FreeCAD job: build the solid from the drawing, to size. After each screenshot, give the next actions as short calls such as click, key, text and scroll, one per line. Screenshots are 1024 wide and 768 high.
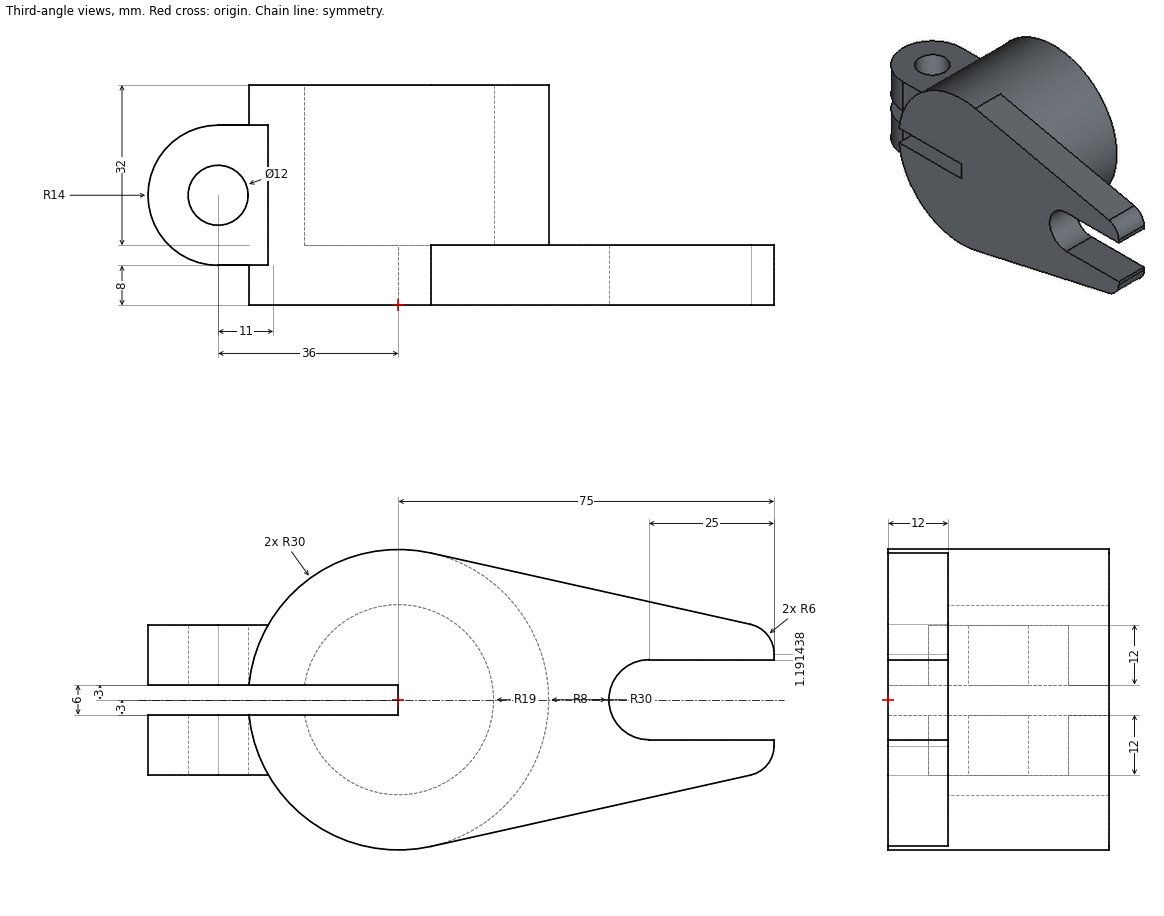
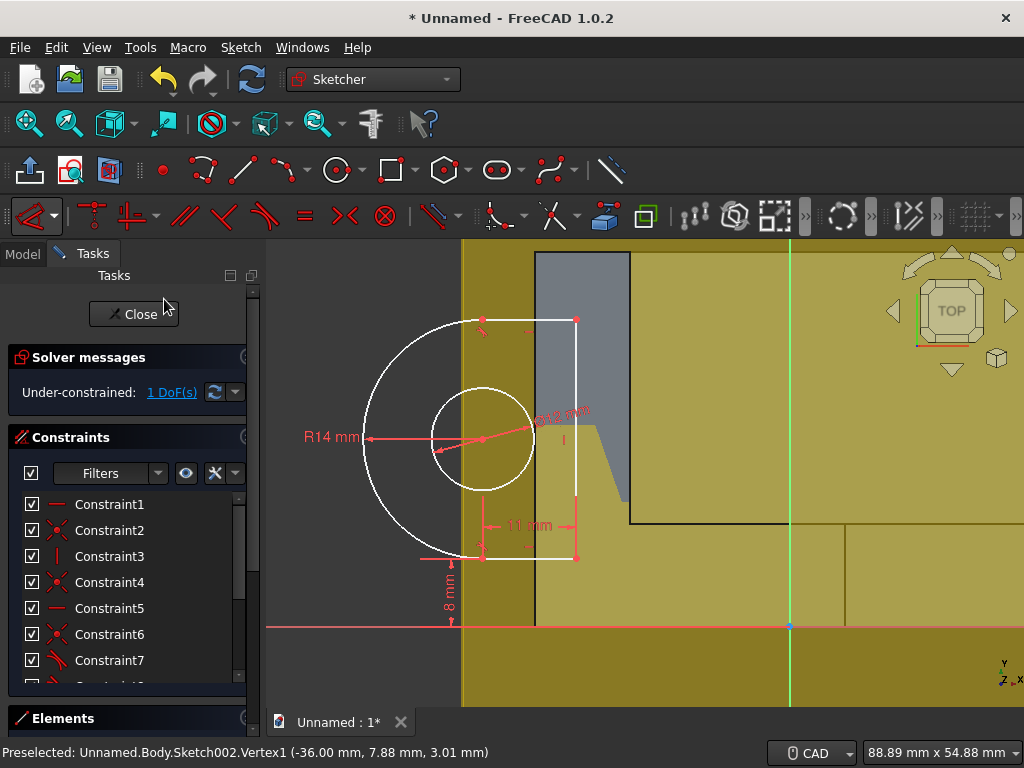
click(483, 439)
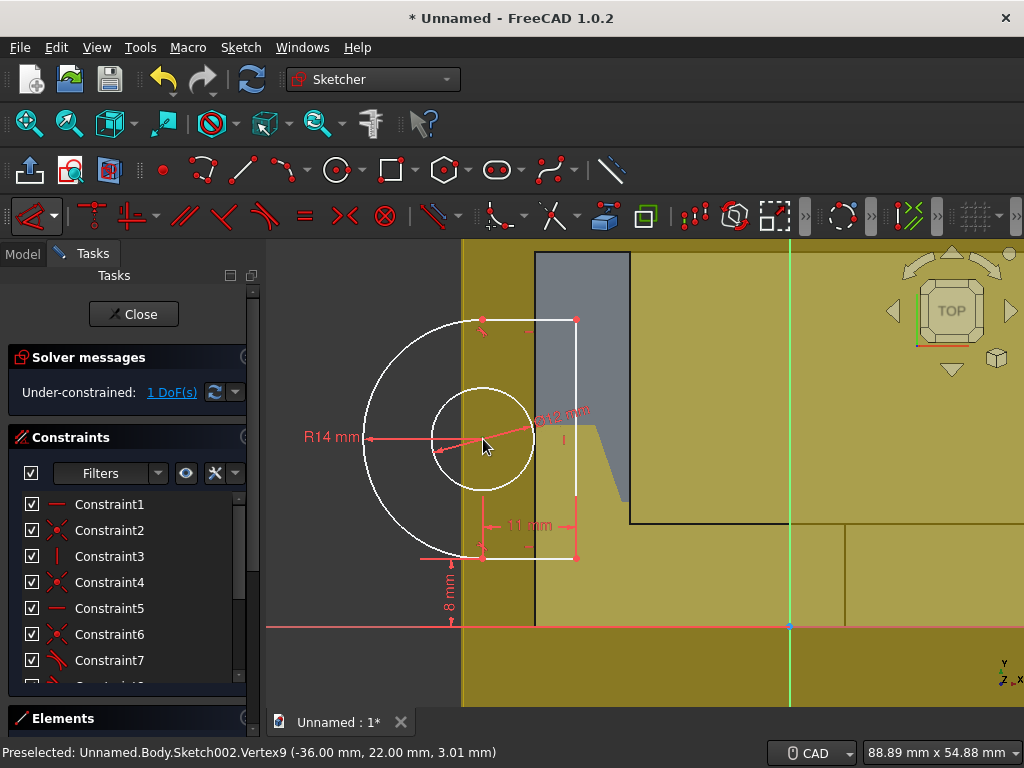
key(l)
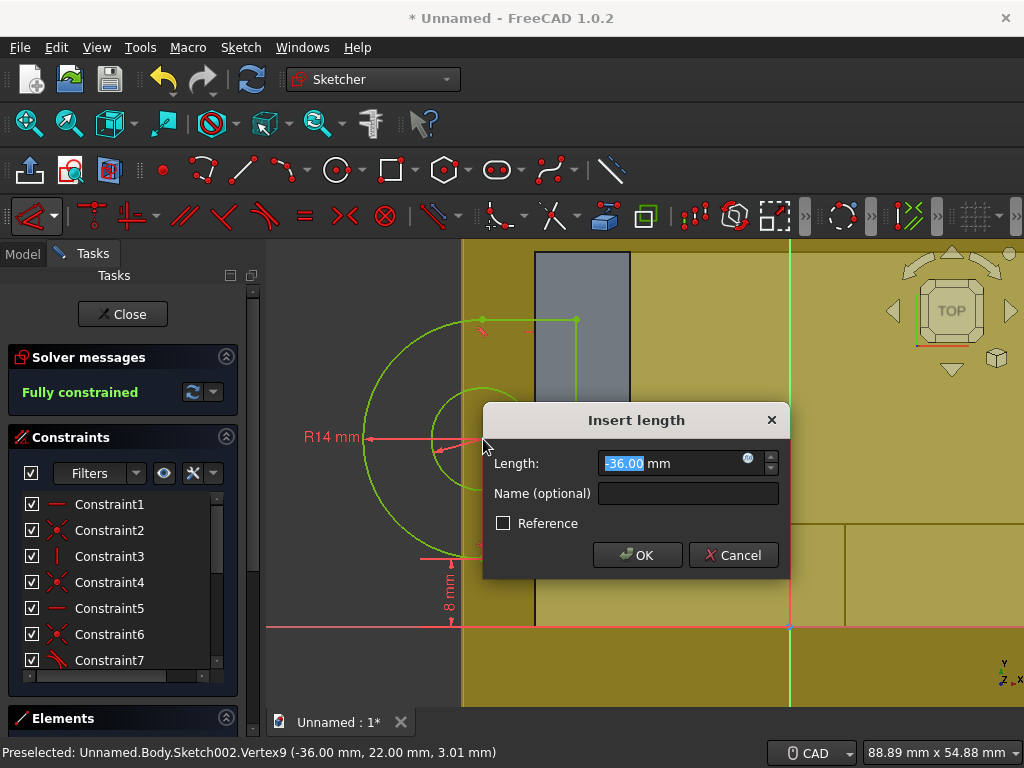
text(-36)
key(Return)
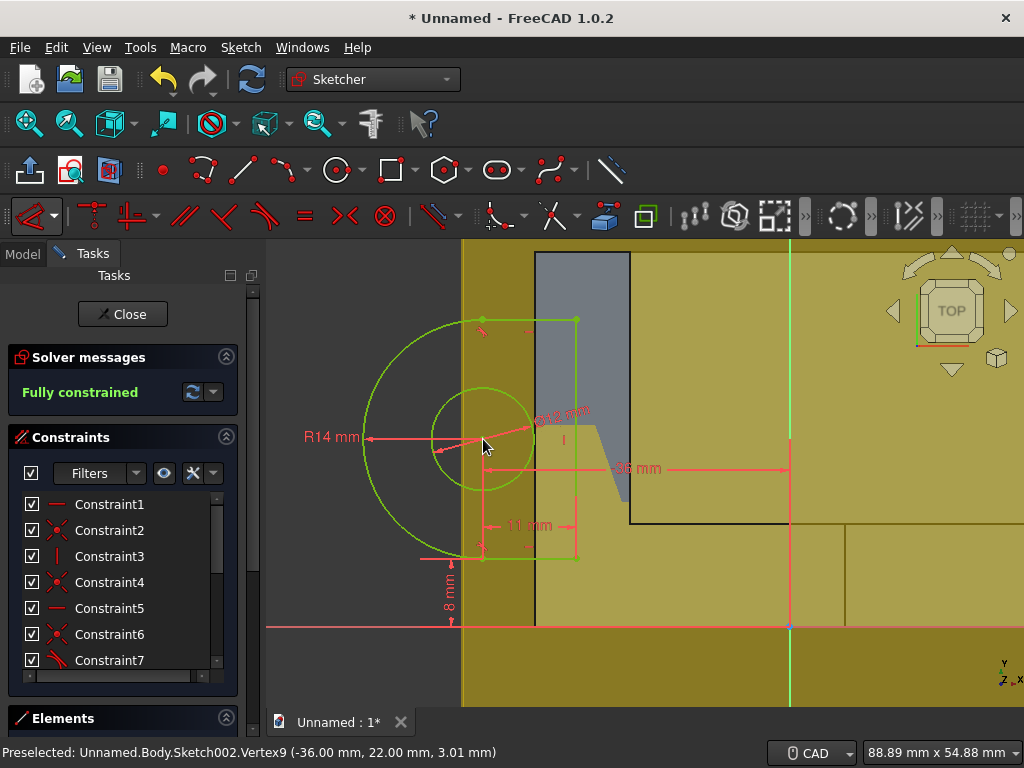
click(123, 314)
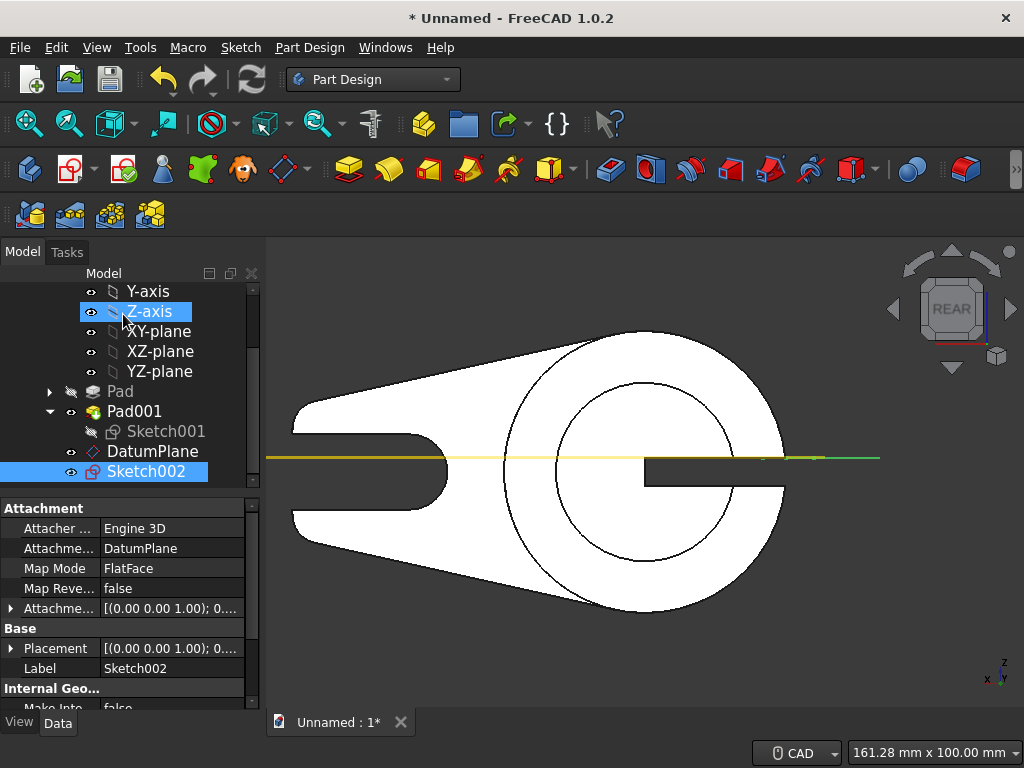
click(350, 170)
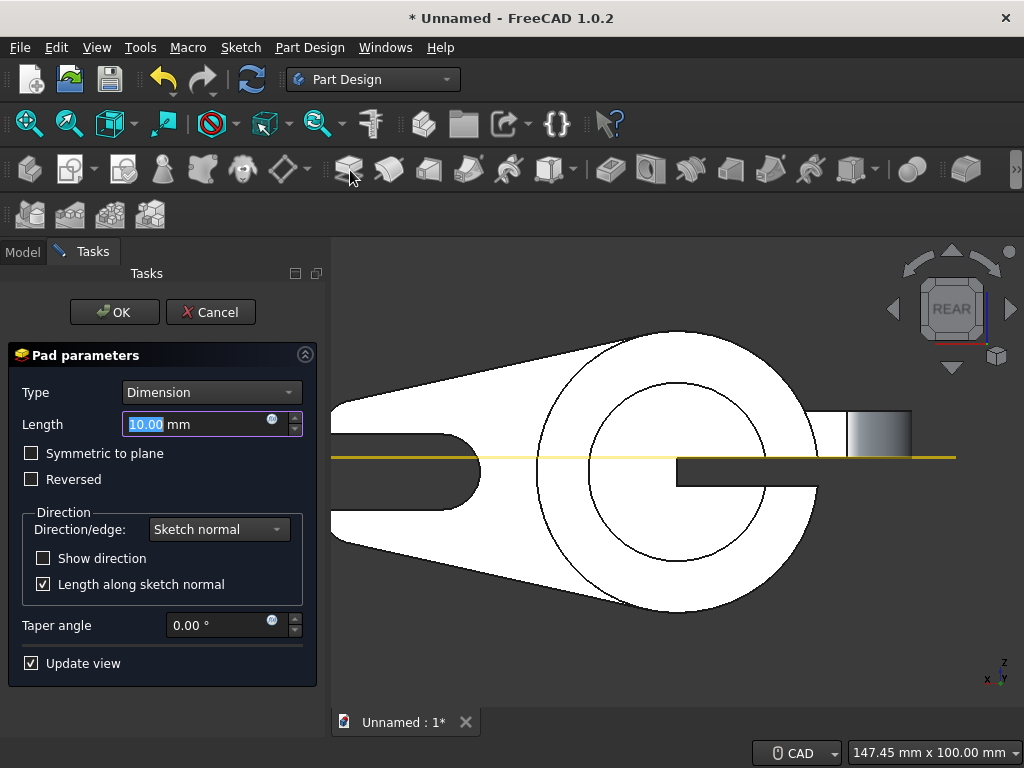
text(12)
key(Tab)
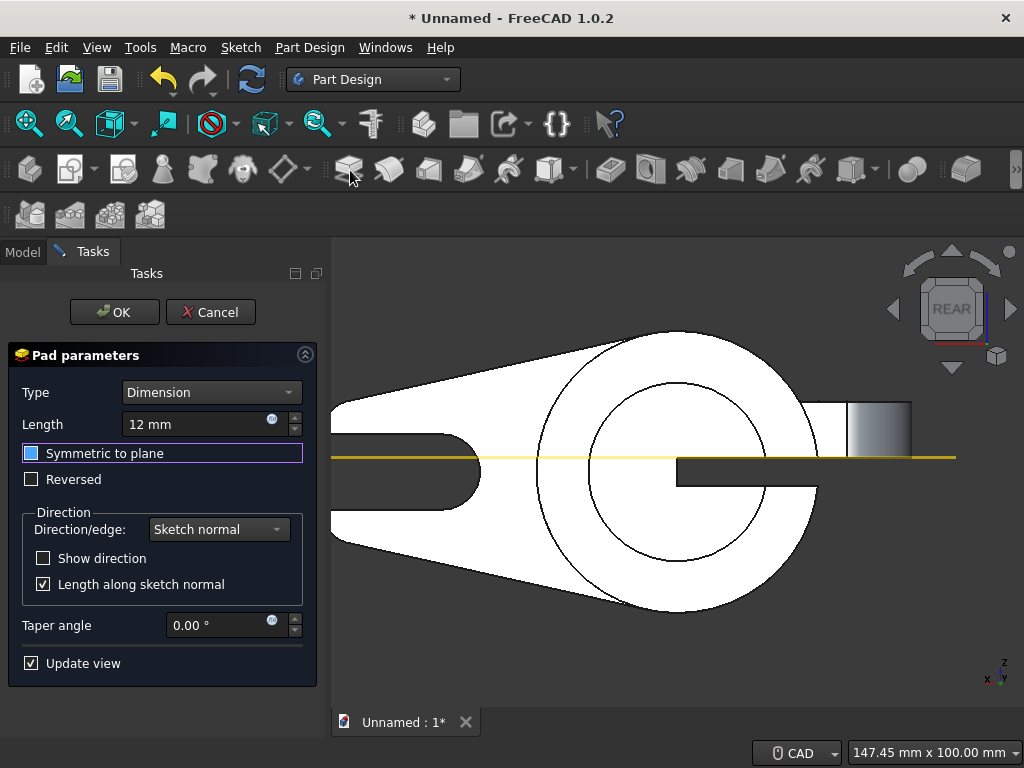
click(115, 312)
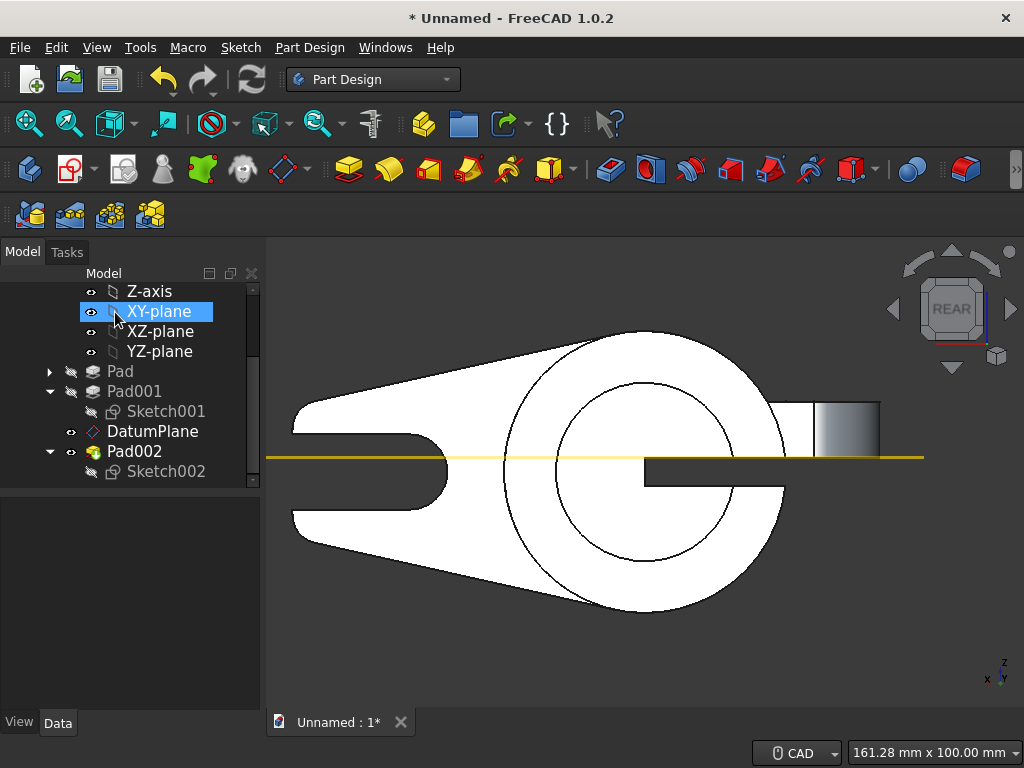
click(116, 432)
key(space)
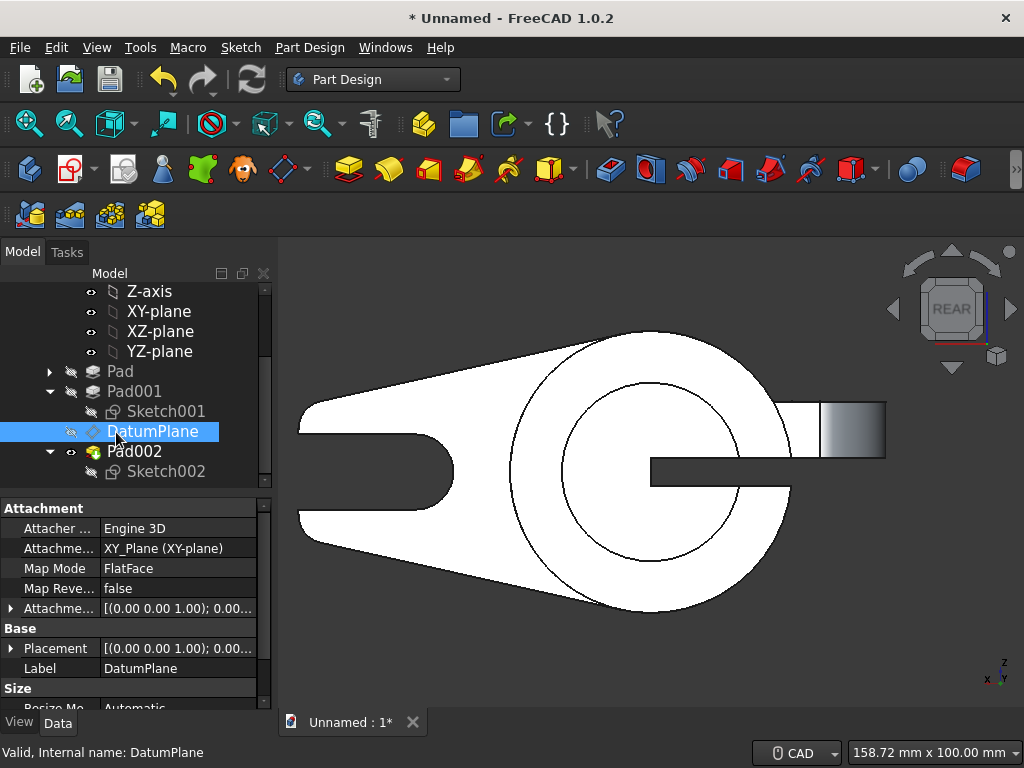
scroll(160, 387, down, 3)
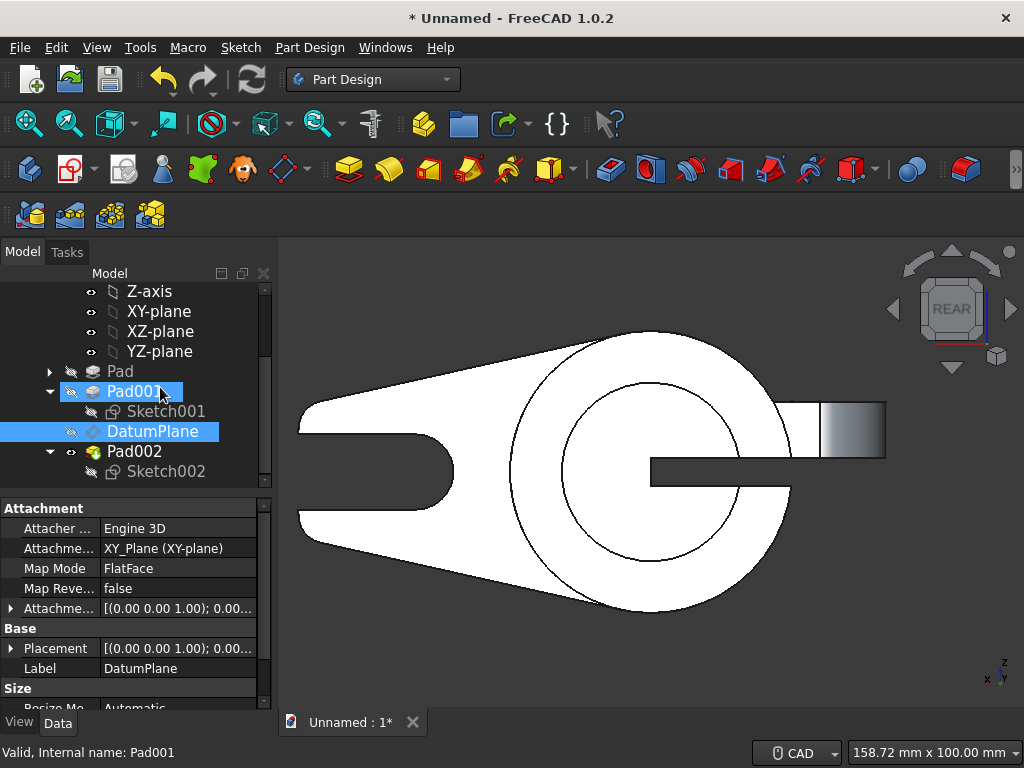
scroll(160, 387, up, 15)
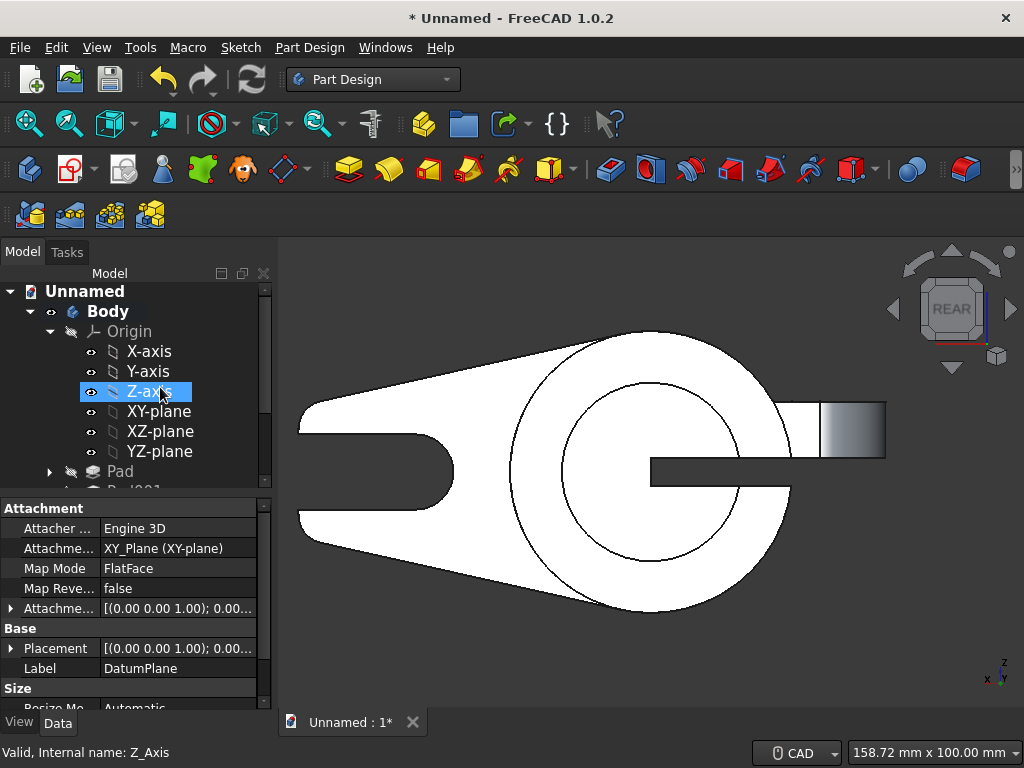
click(136, 412)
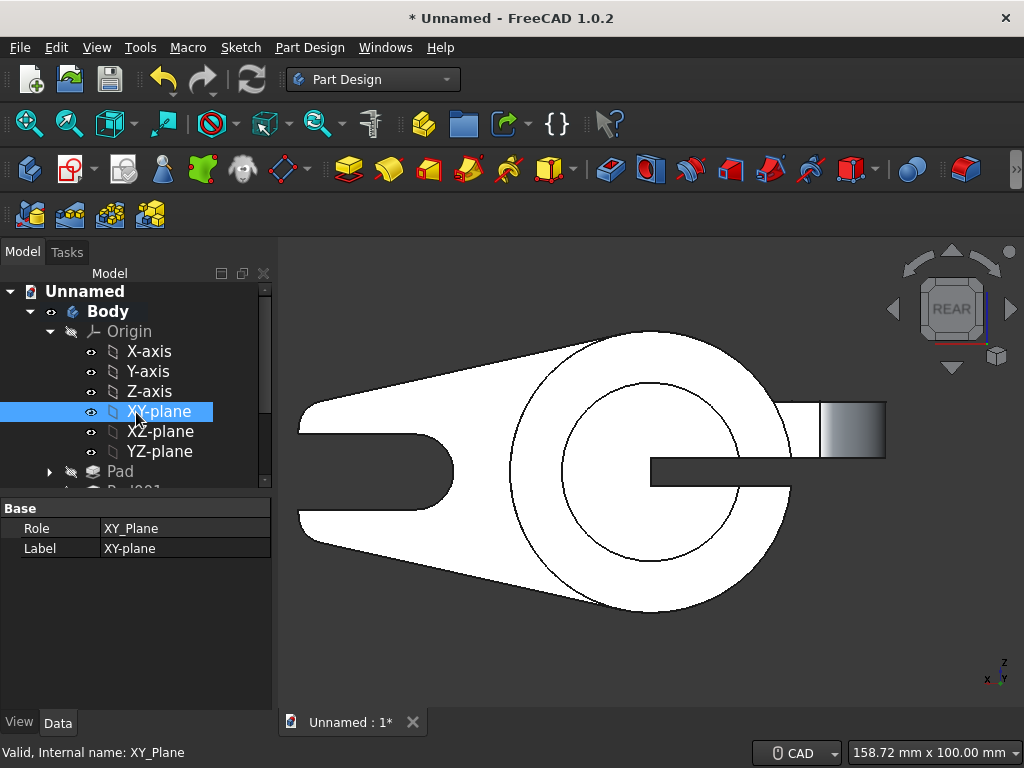
click(284, 170)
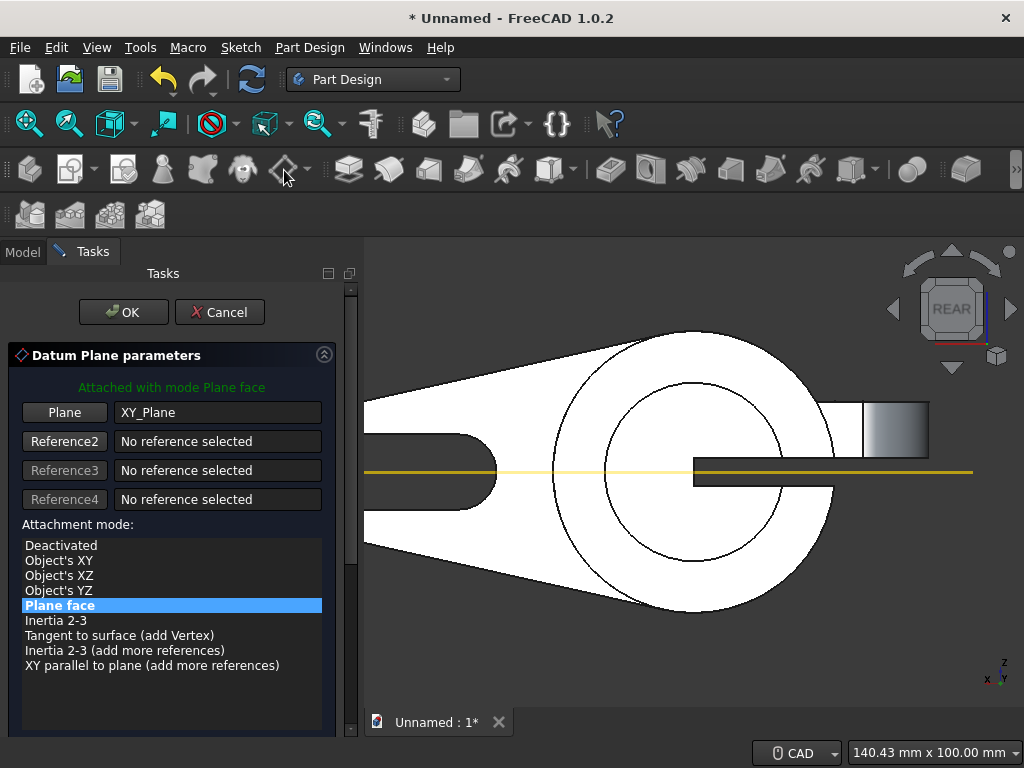
scroll(351, 510, down, 3)